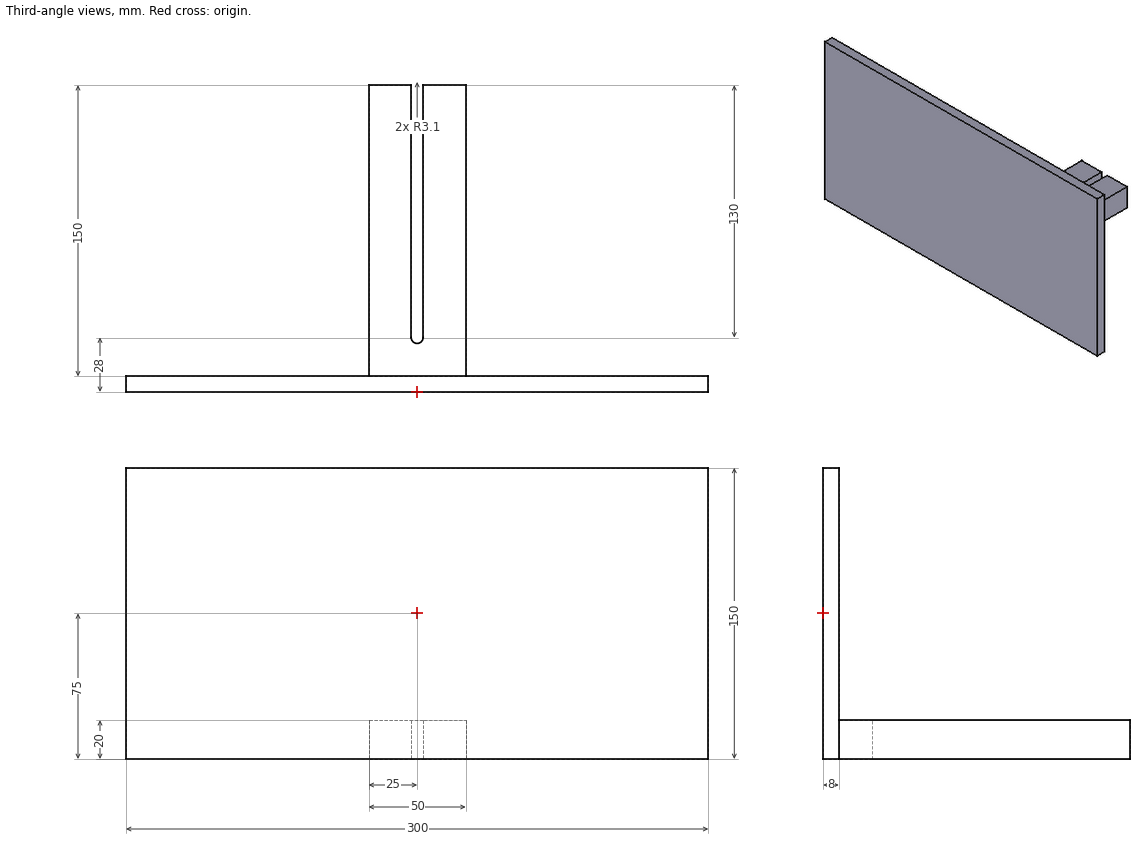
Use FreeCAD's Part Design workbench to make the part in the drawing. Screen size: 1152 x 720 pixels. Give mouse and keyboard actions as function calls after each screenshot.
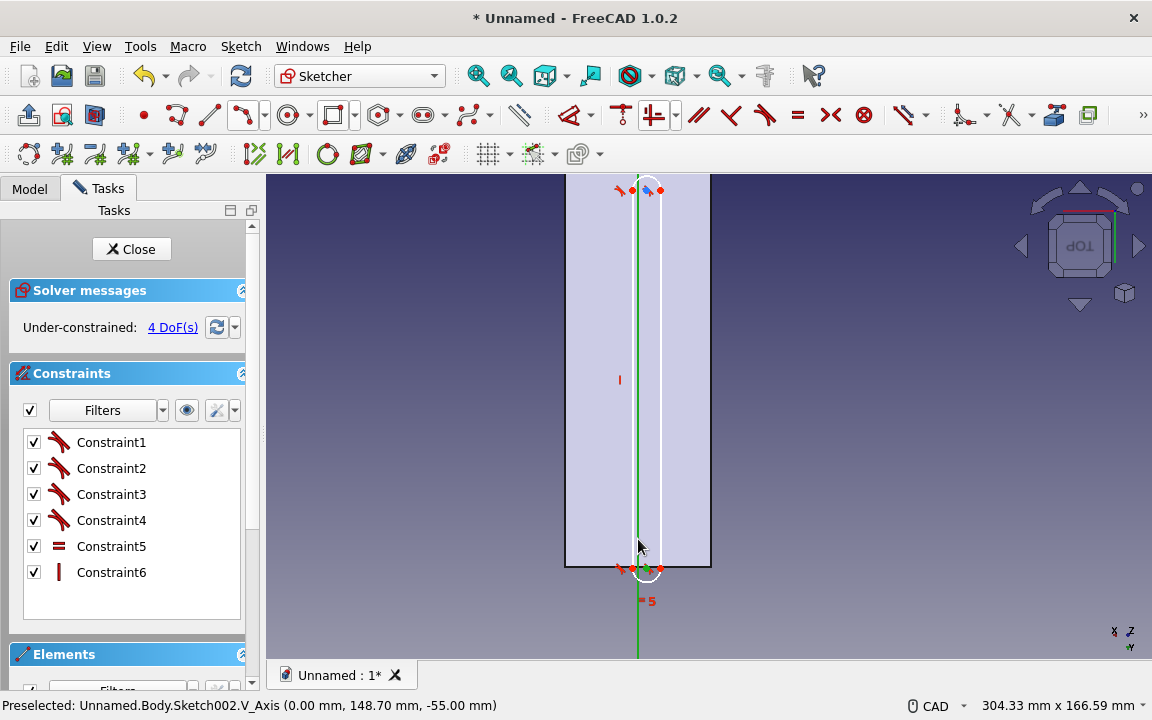
click(621, 116)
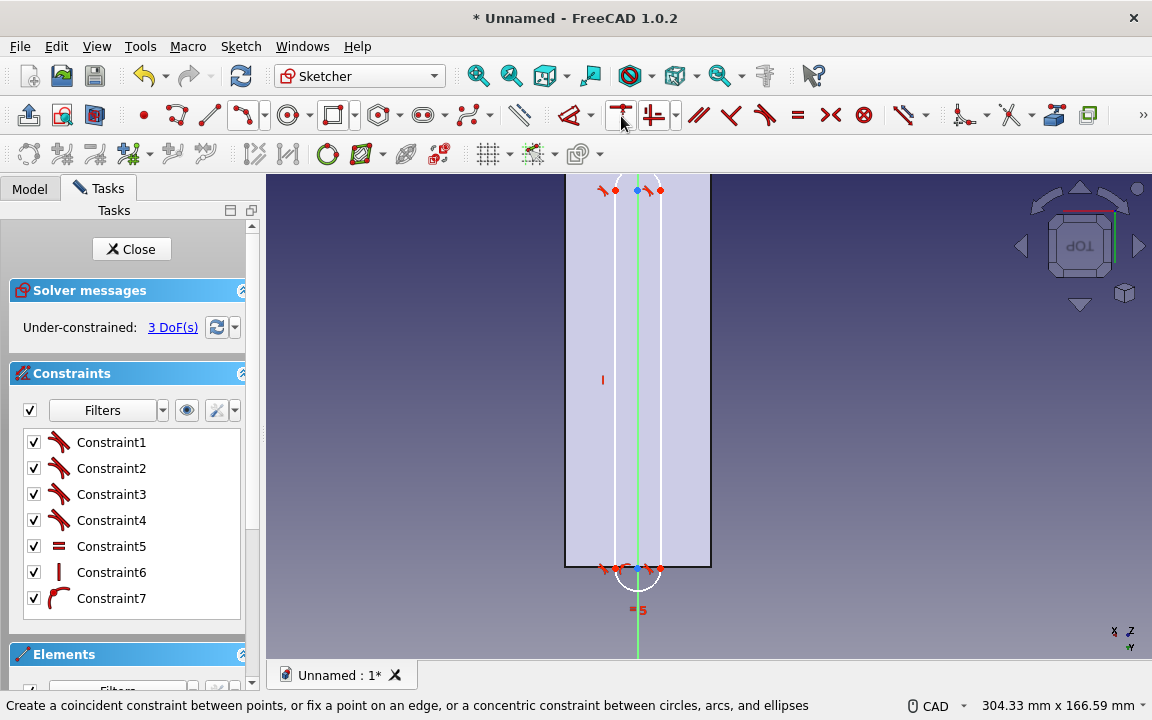
click(568, 116)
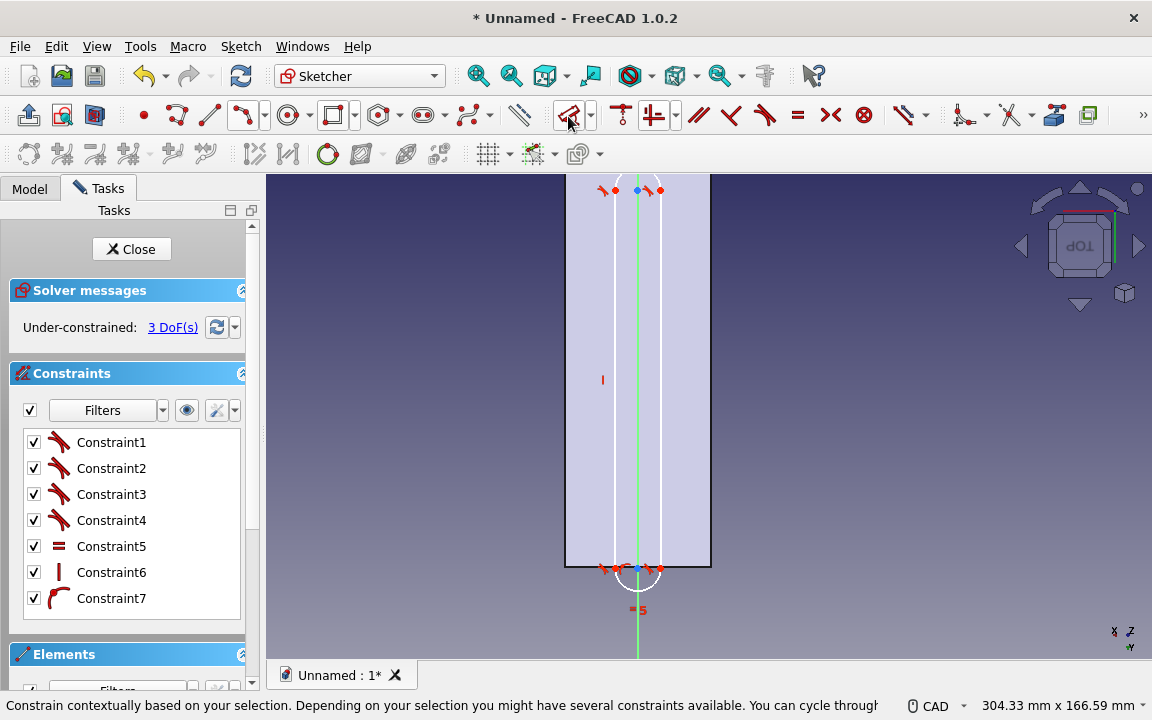
scroll(625, 587, up, 8)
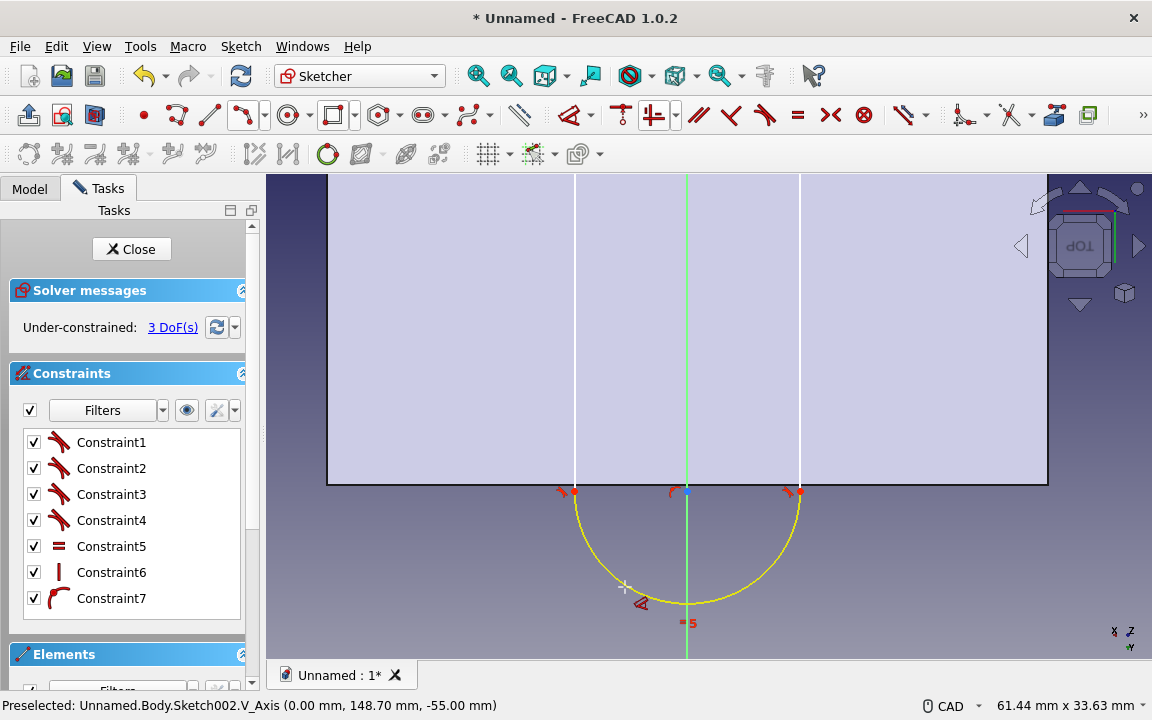
click(621, 582)
click(602, 608)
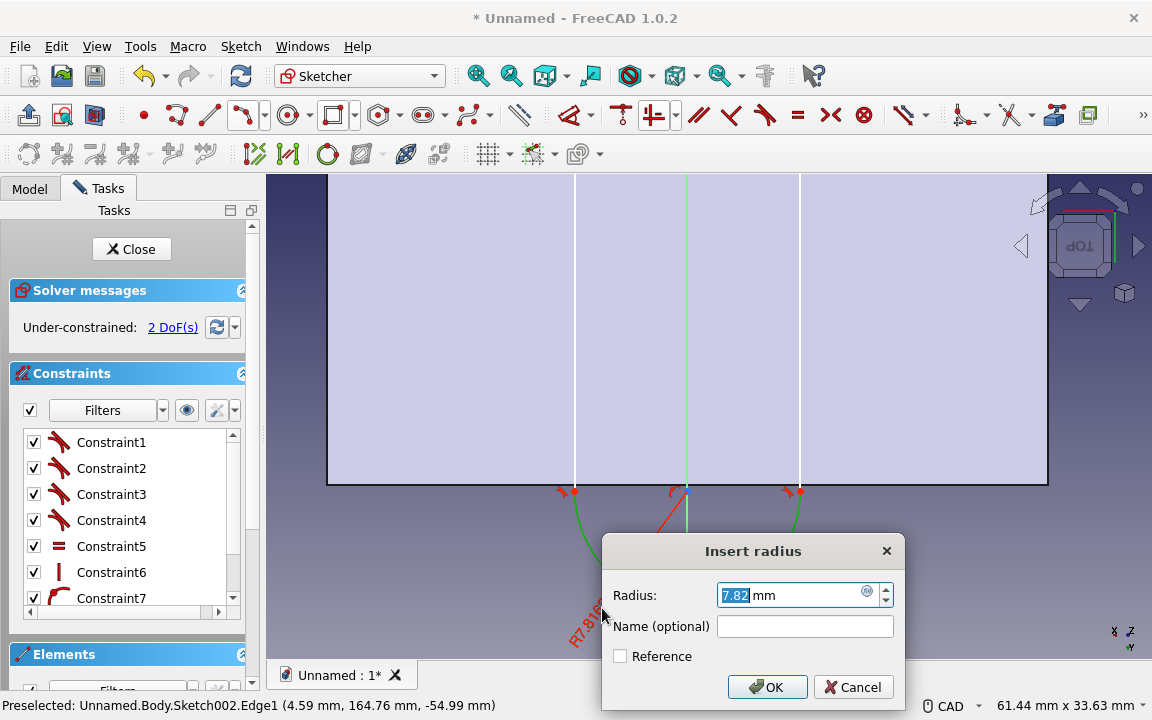
text(3.1)
key(Return)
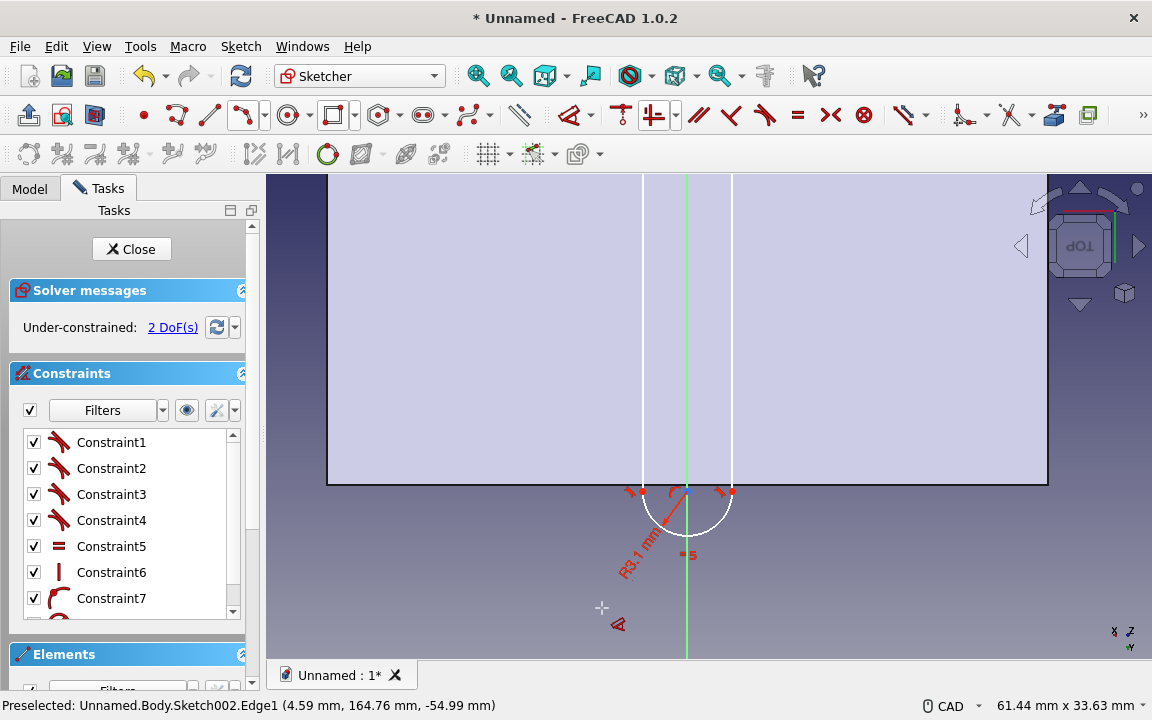
scroll(633, 581, down, 10)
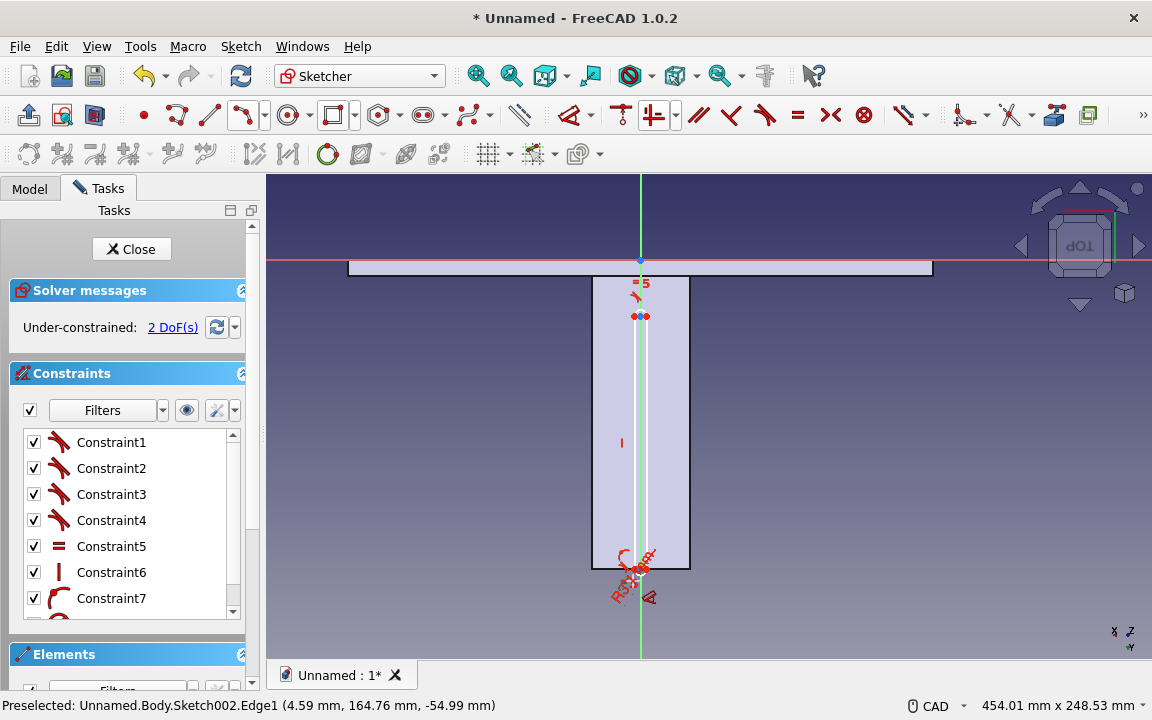
scroll(635, 494, up, 5)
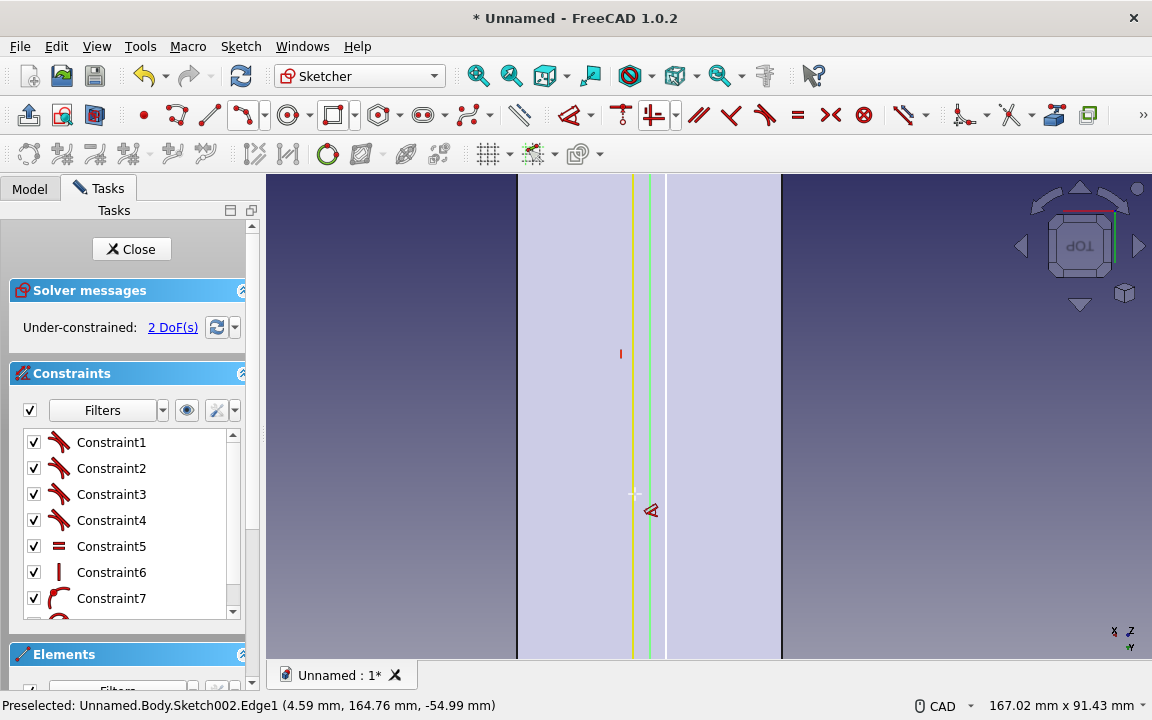
click(633, 492)
click(599, 416)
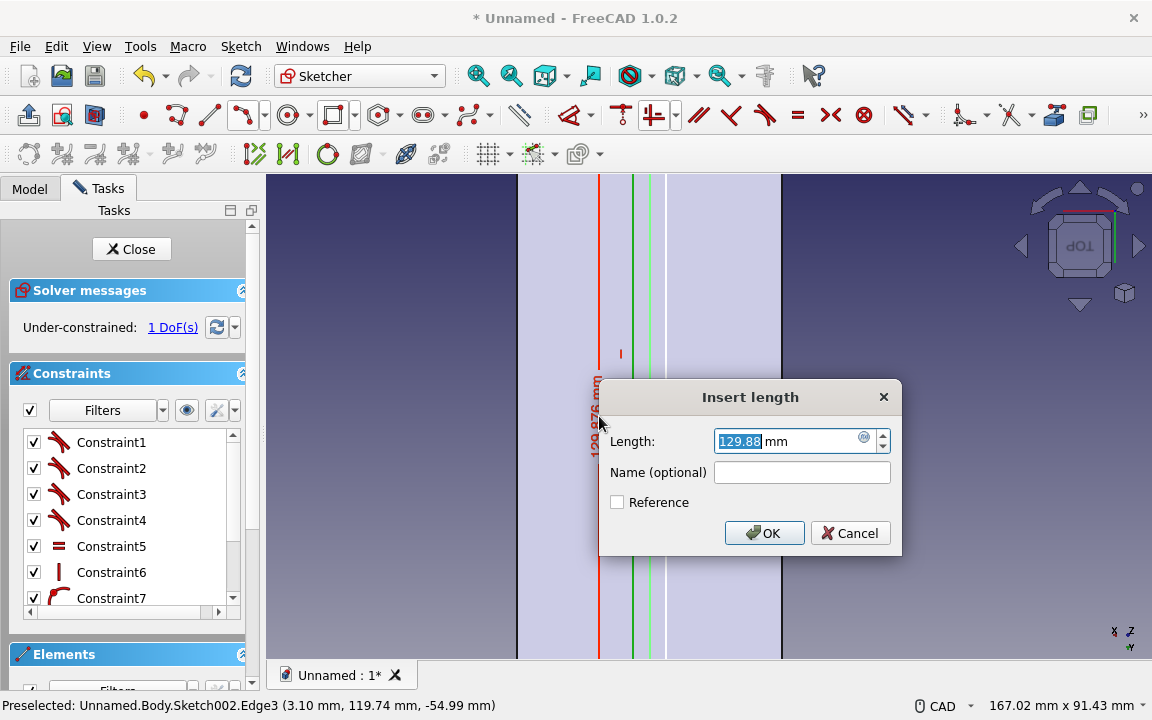
text(130)
key(Return)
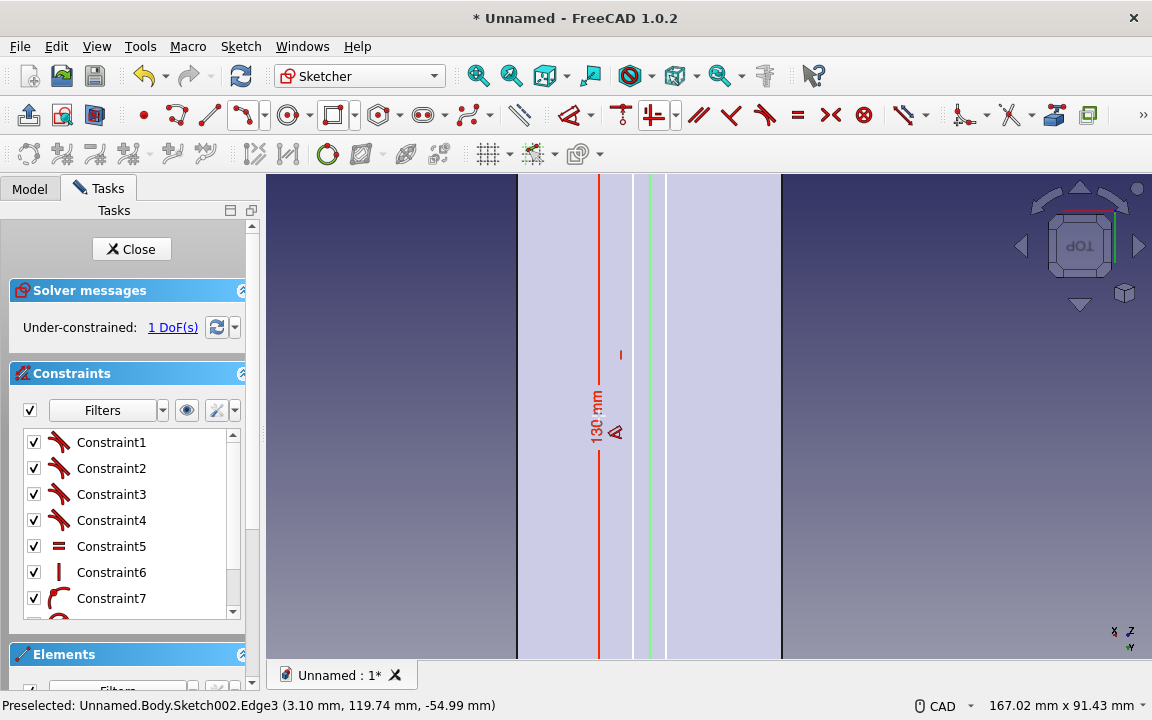
scroll(635, 493, down, 5)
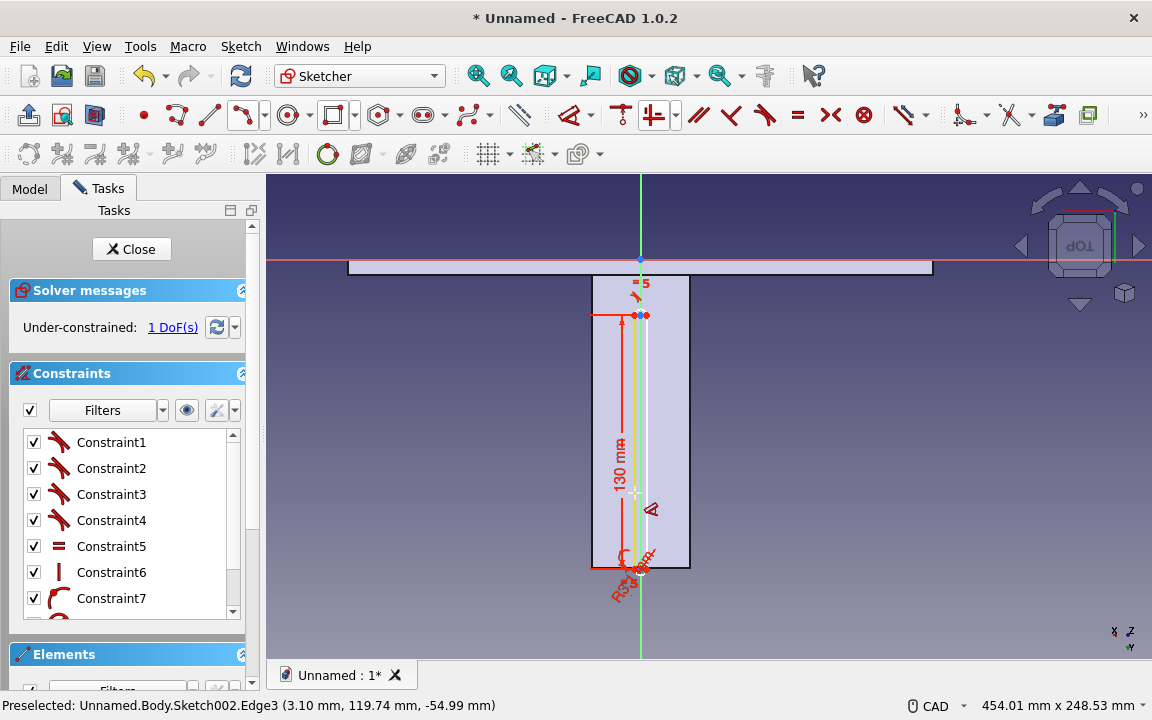
scroll(647, 315, up, 4)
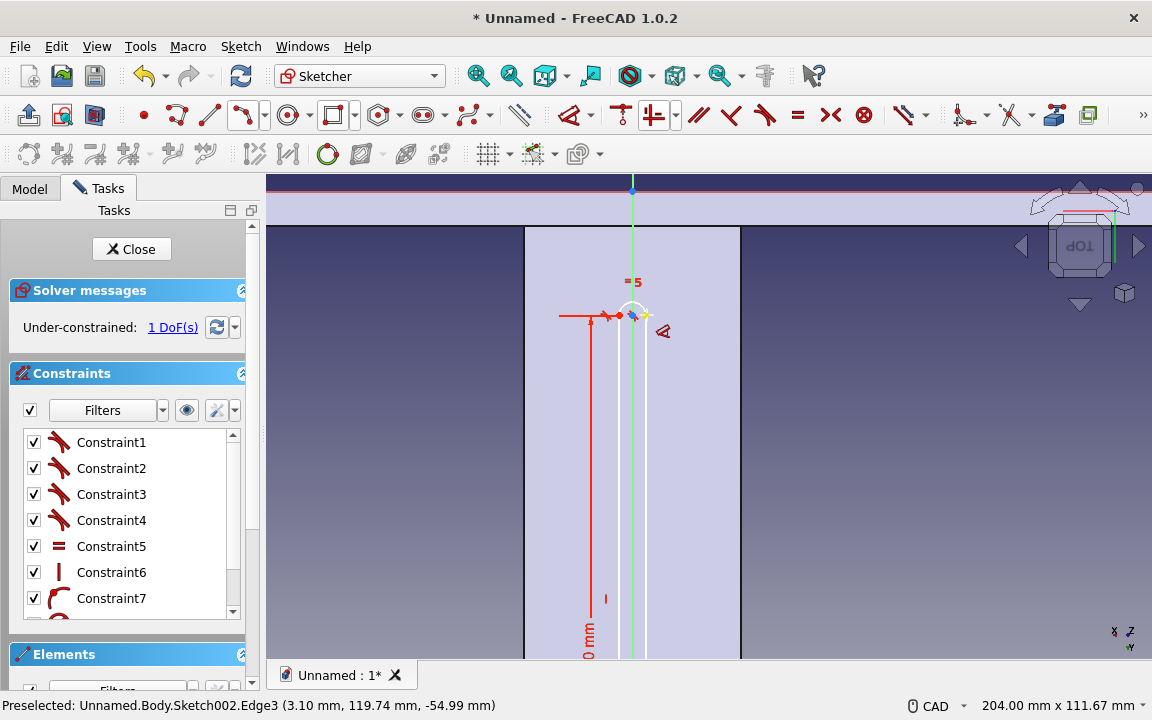
click(646, 316)
click(680, 259)